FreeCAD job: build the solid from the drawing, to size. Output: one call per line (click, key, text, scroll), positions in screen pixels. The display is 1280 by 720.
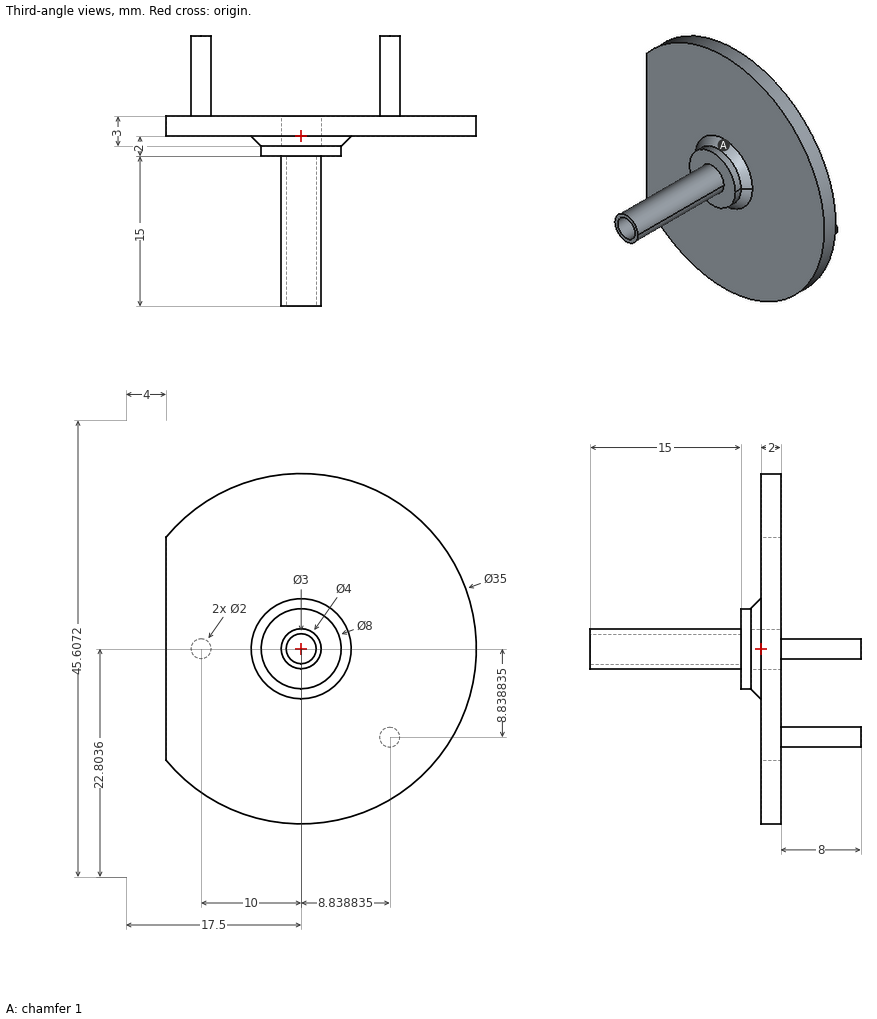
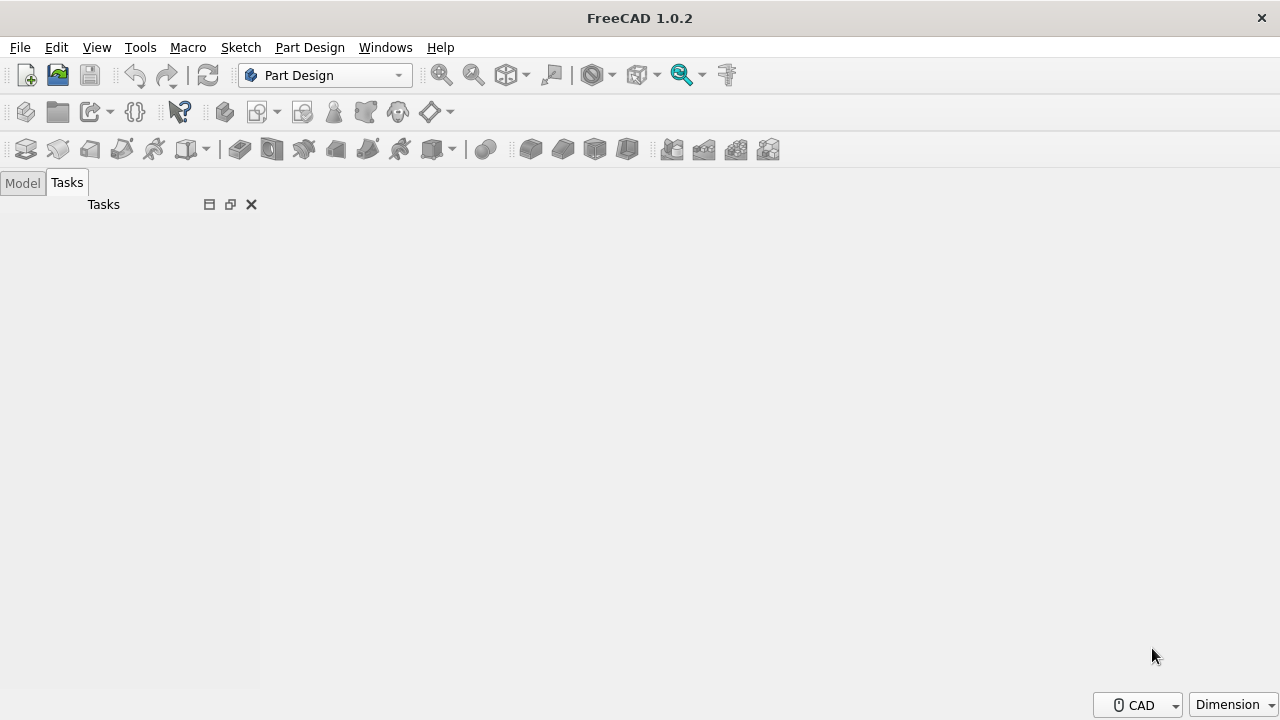
click(26, 76)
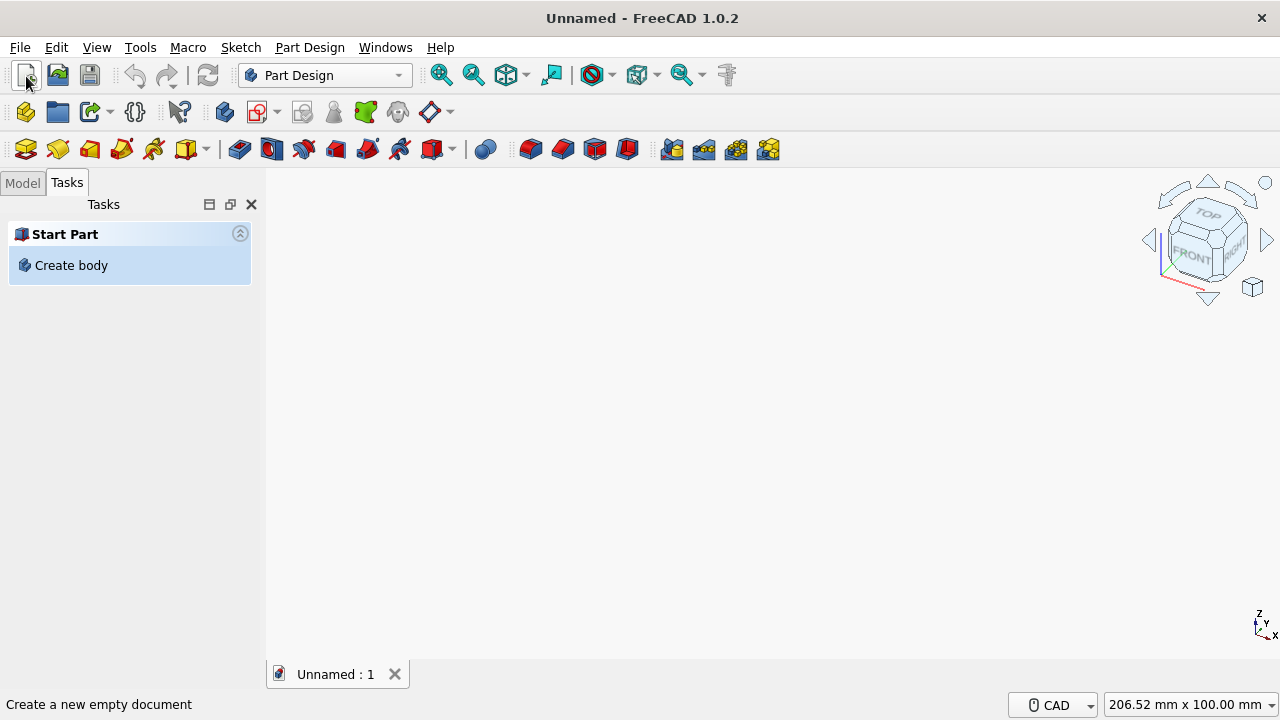
click(258, 112)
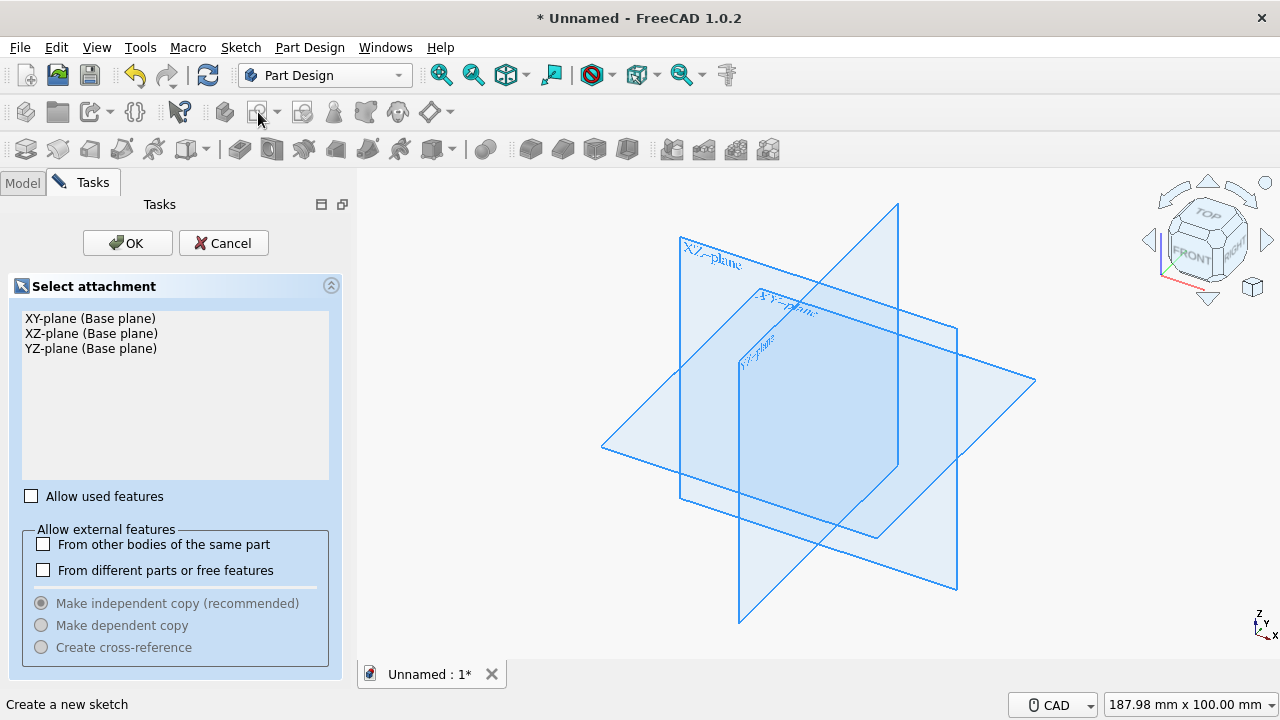
click(82, 334)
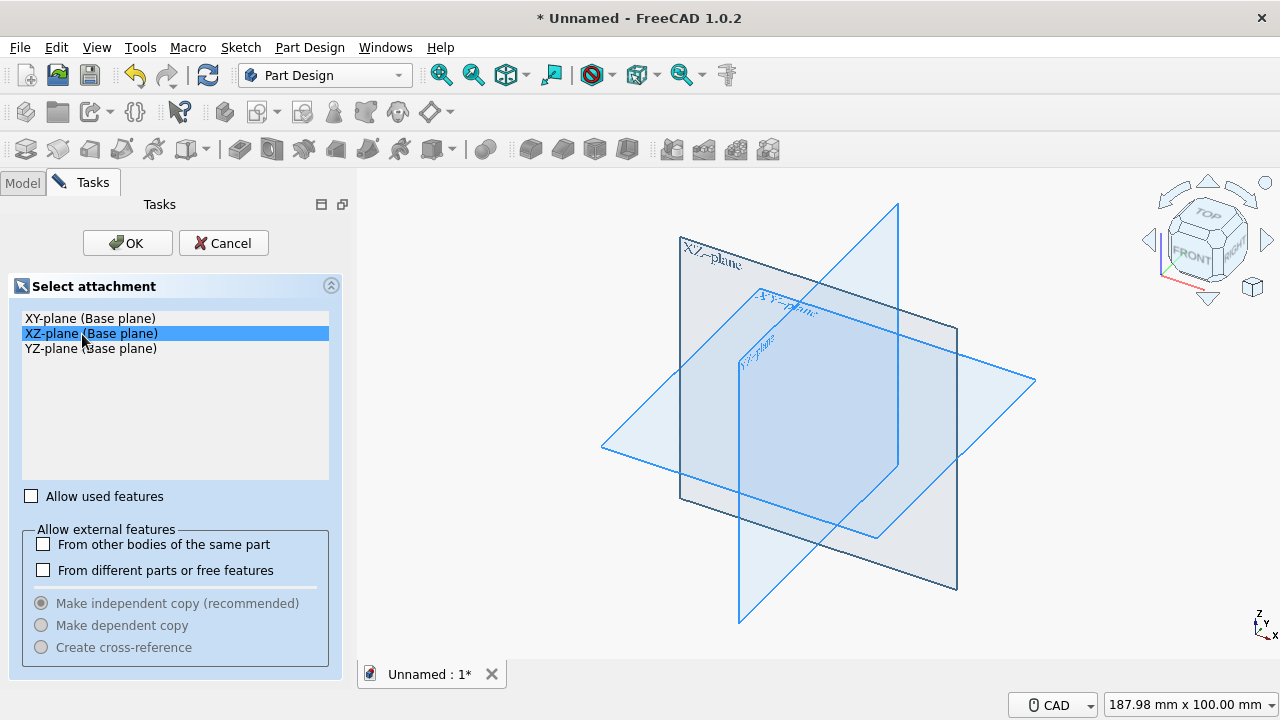
click(128, 243)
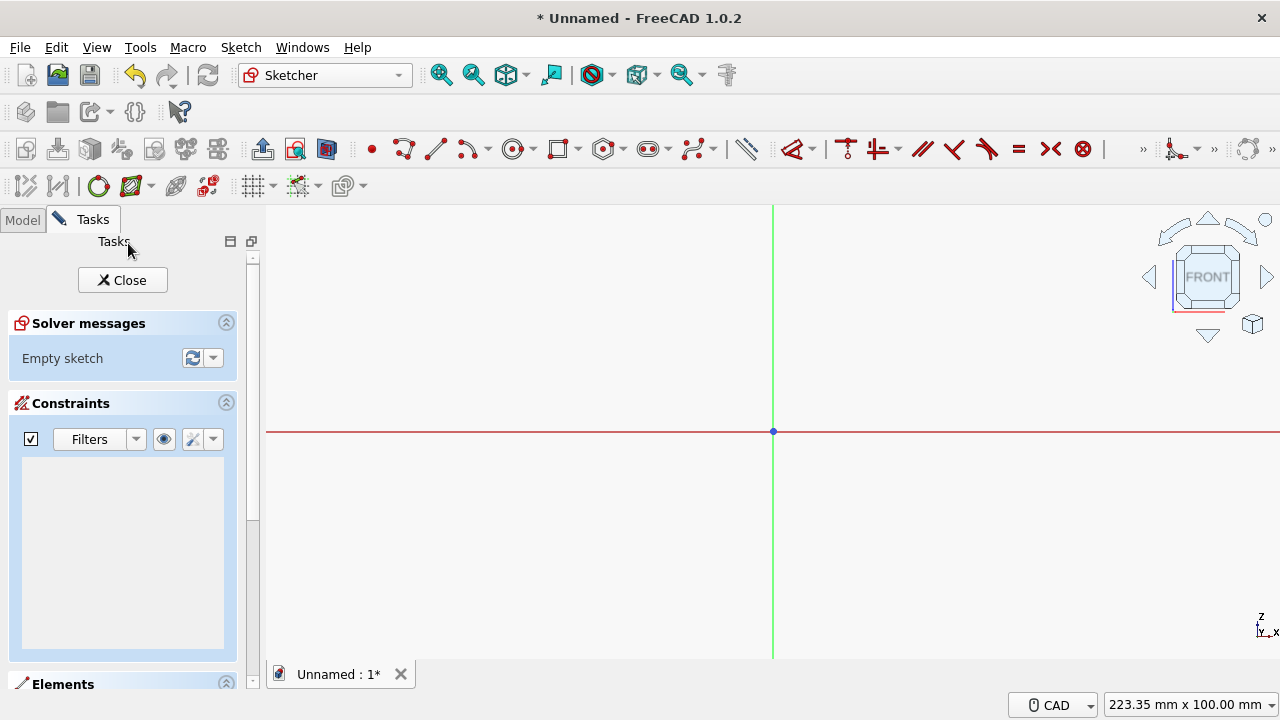
scroll(856, 432, up, 3)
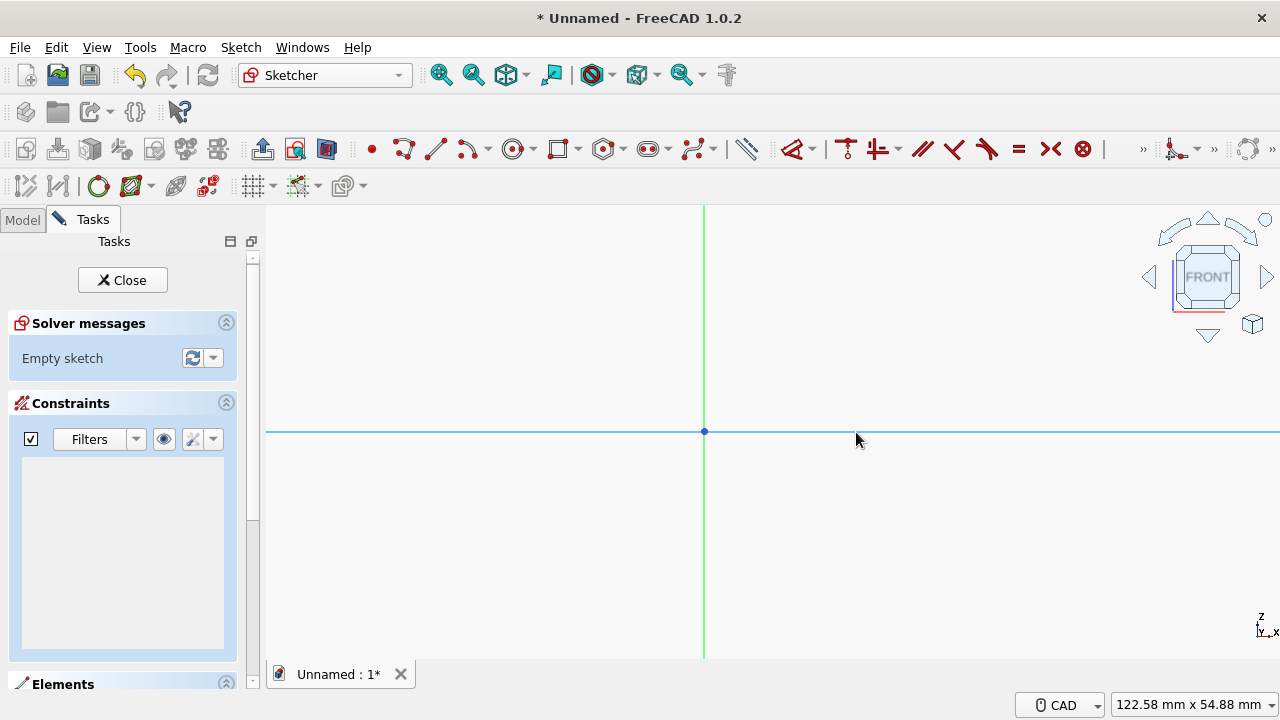
click(514, 150)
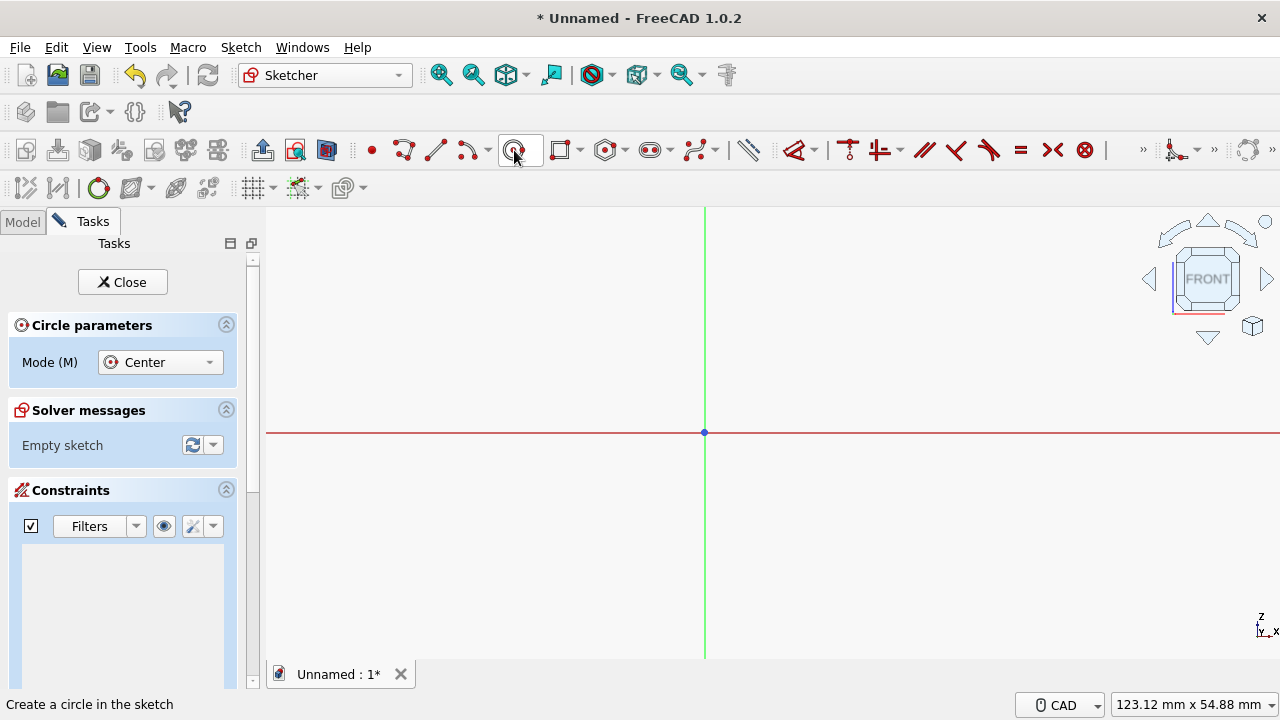
click(705, 433)
click(807, 331)
key(Escape)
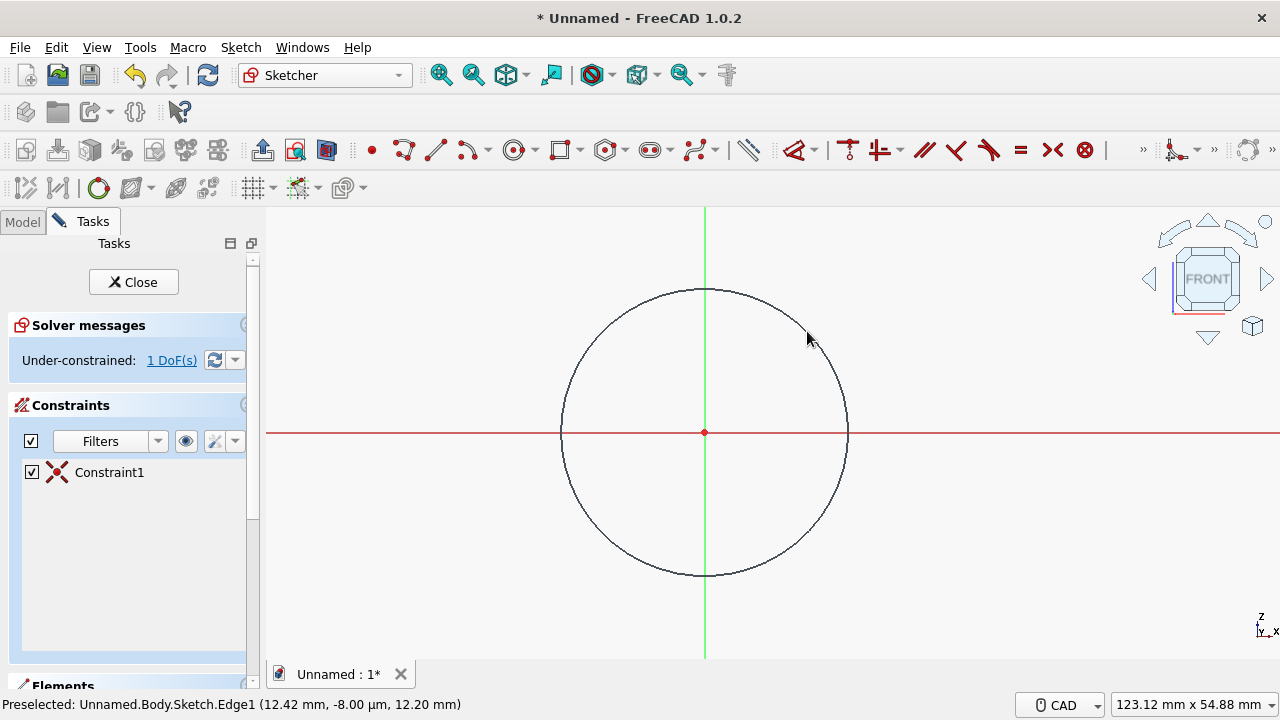
click(794, 150)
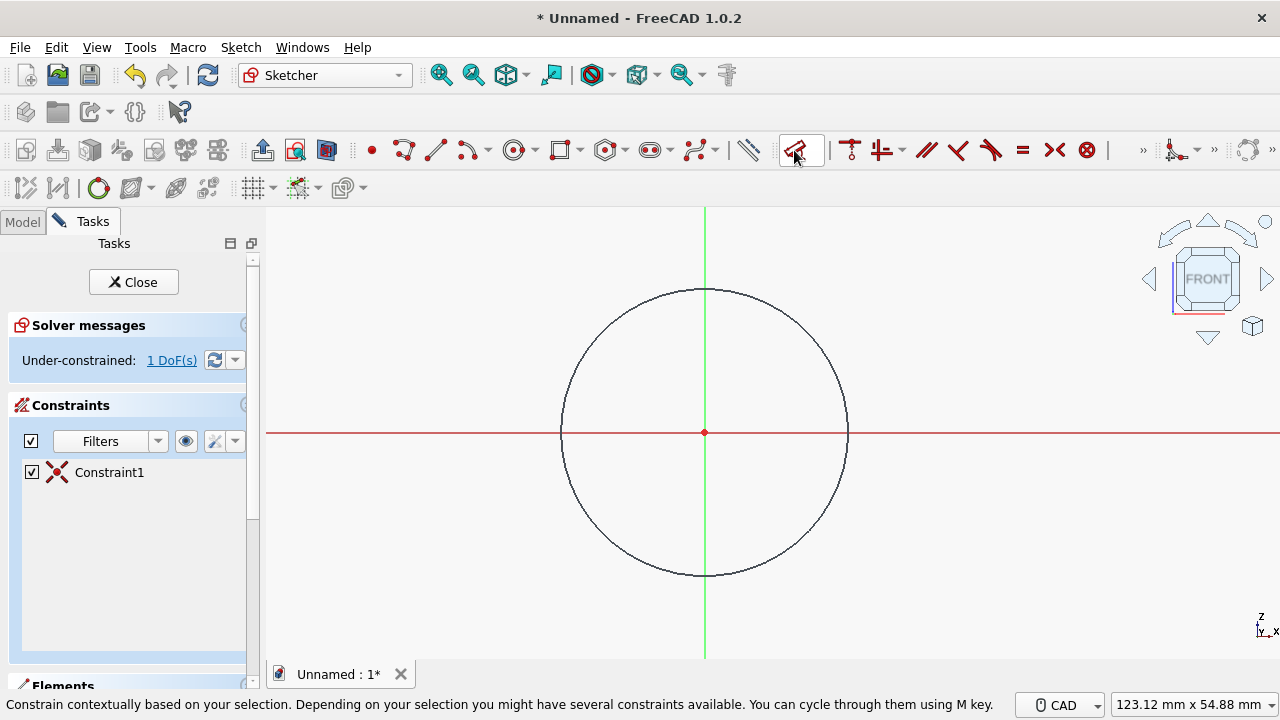
click(806, 331)
click(829, 308)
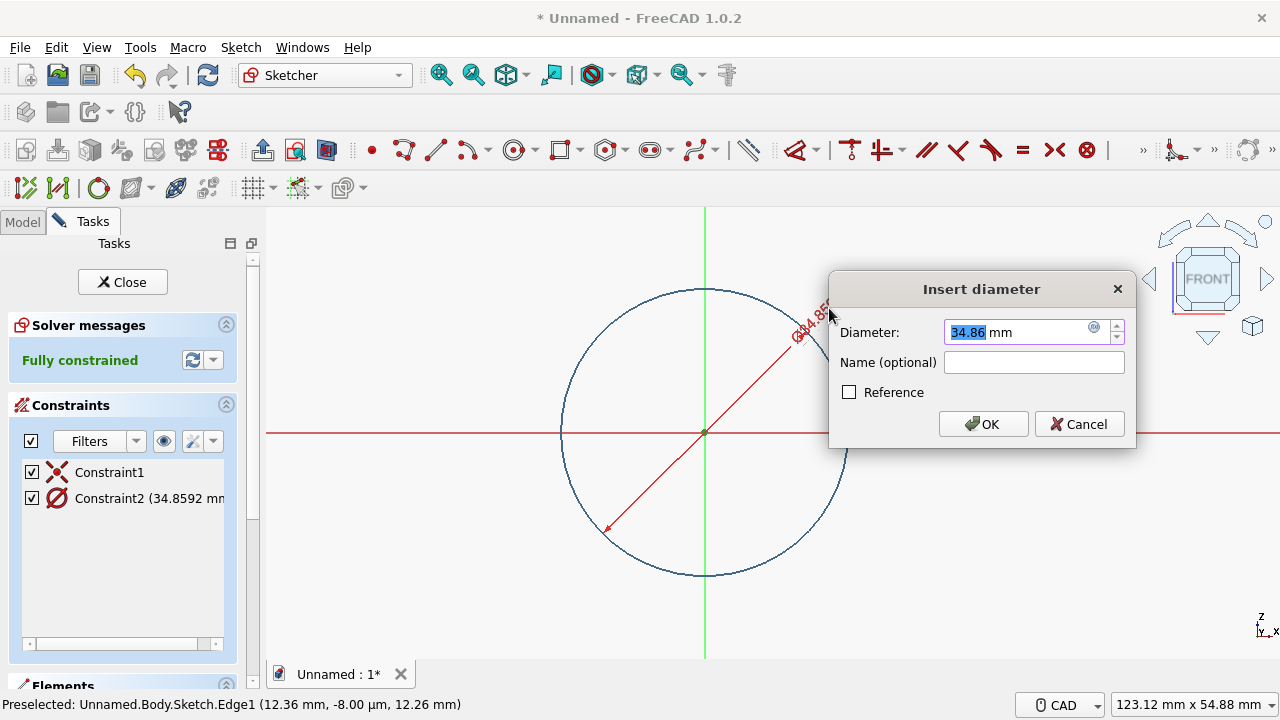
text(35)
key(Return)
key(Escape)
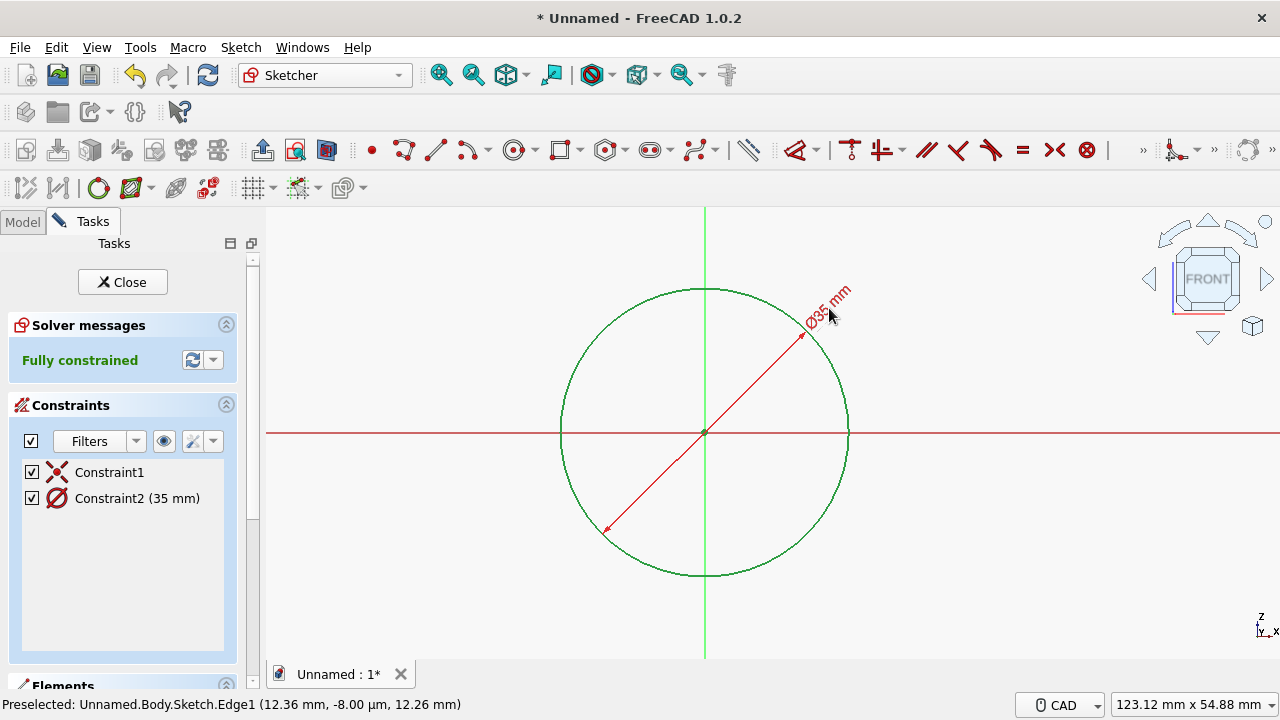
click(123, 282)